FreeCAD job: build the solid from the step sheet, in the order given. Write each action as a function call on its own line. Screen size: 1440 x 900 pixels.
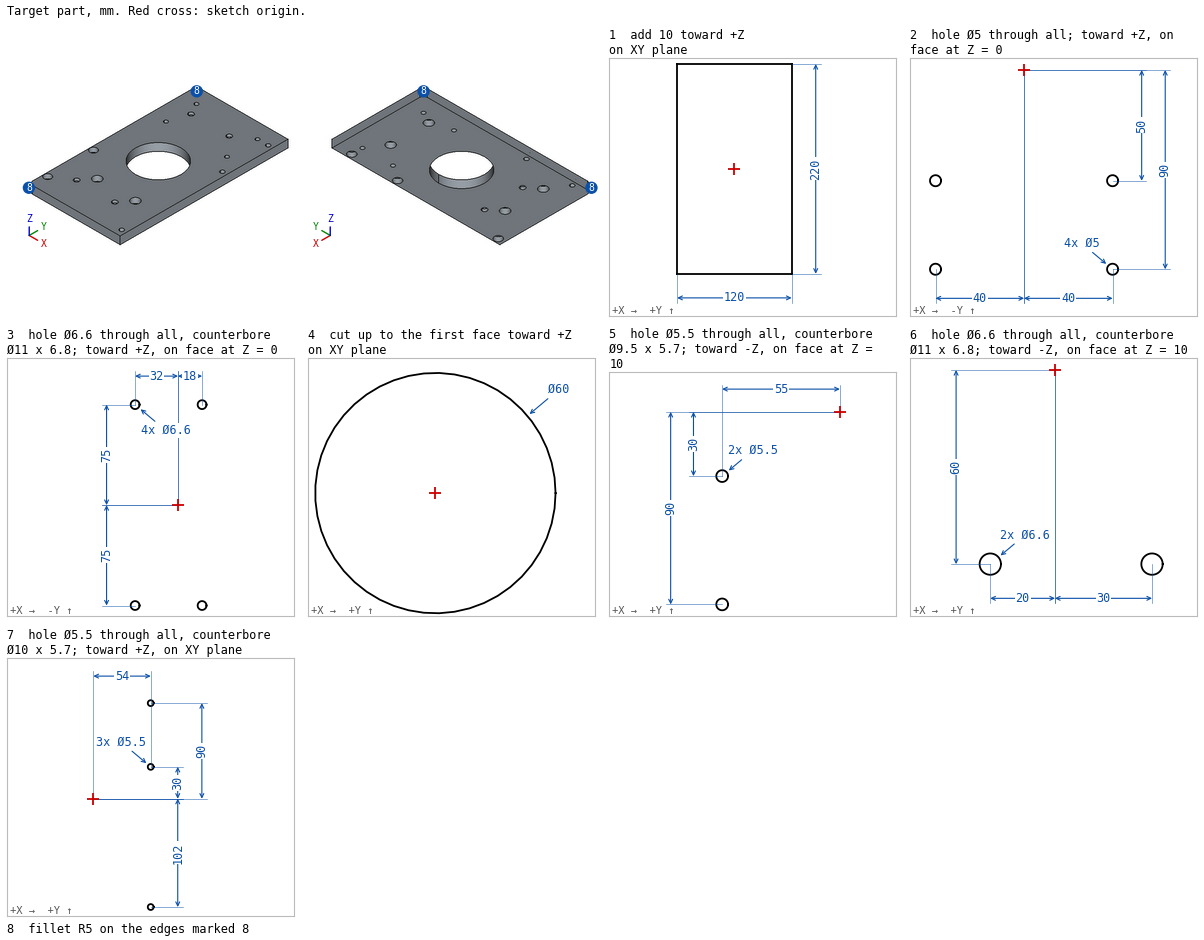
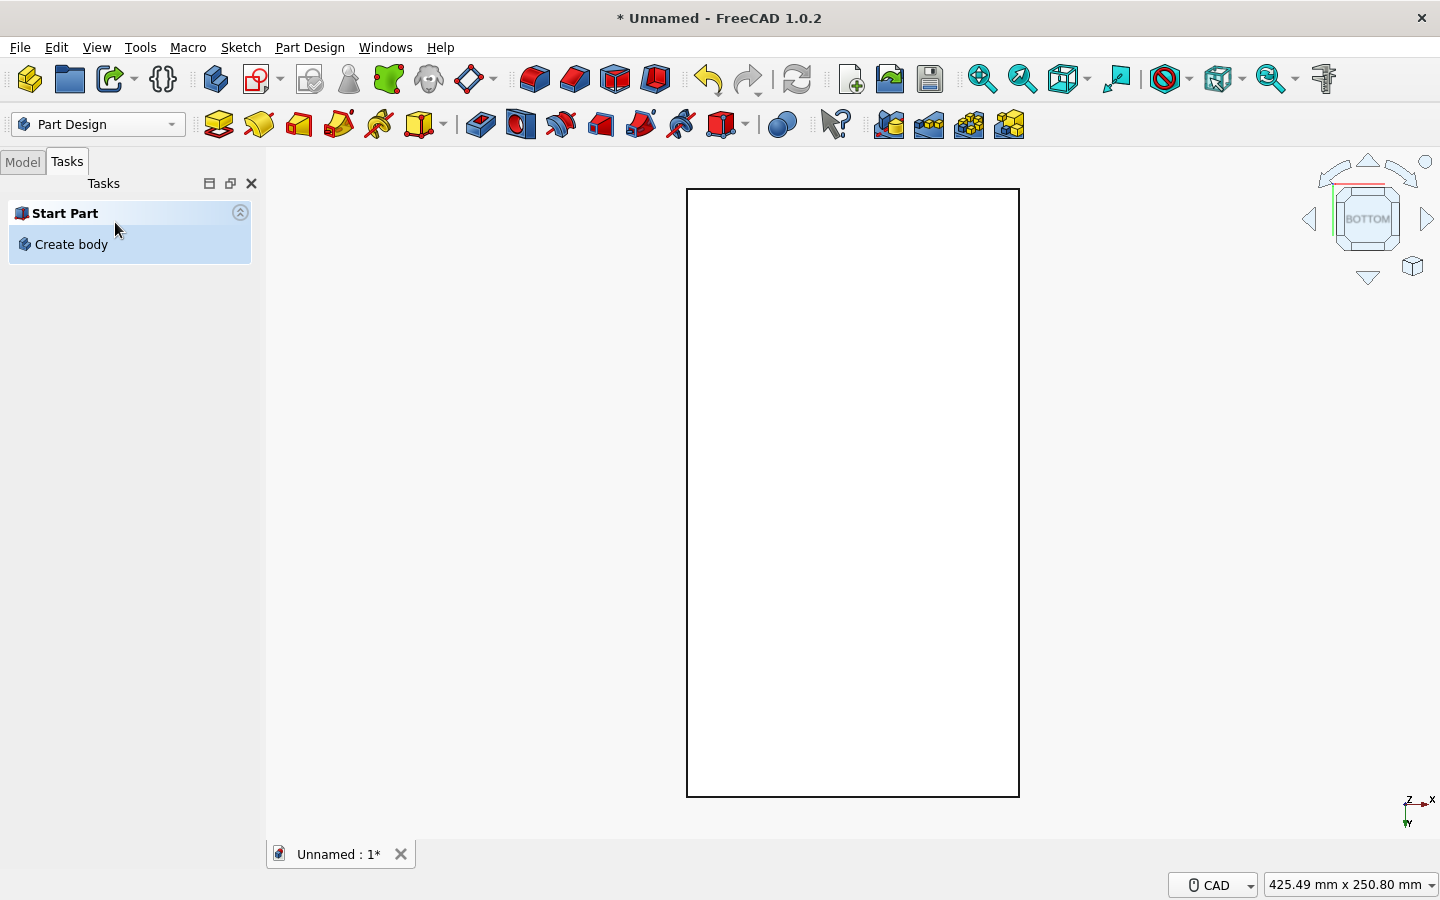
click(853, 579)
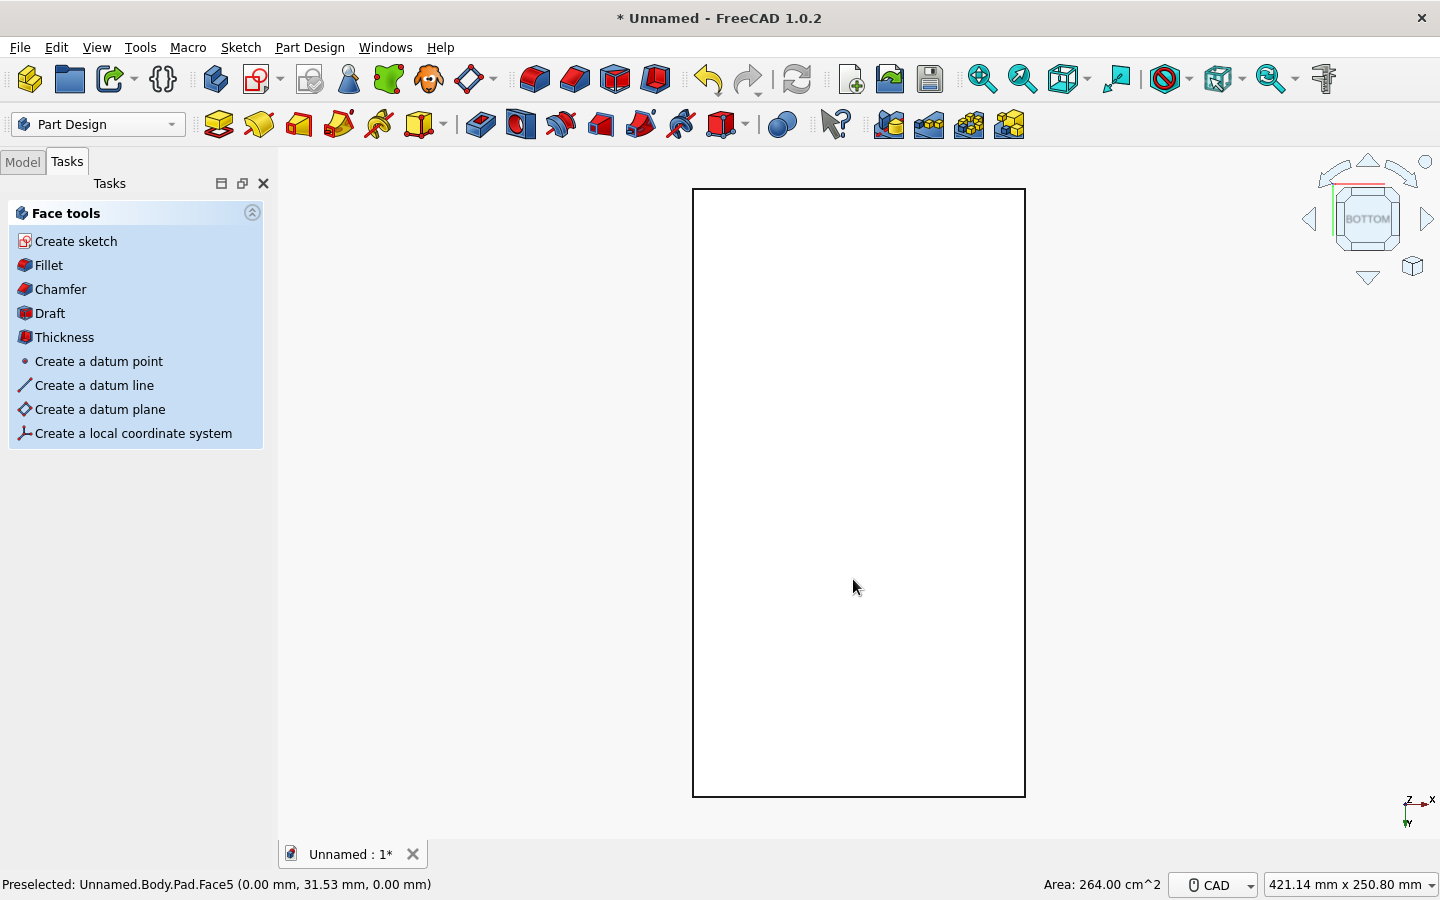
click(256, 80)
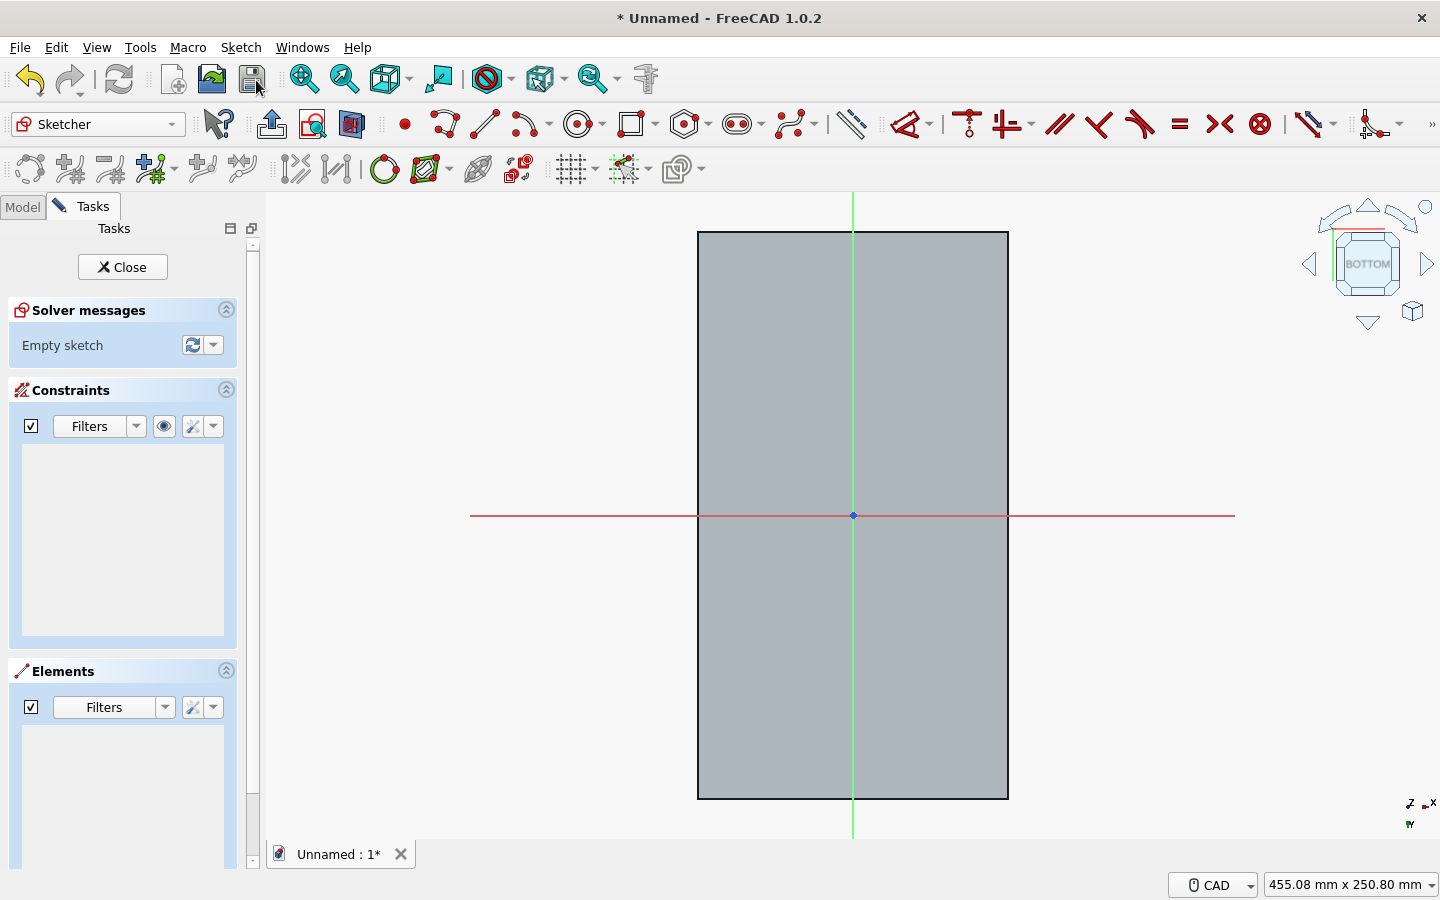
scroll(936, 780, up, 3)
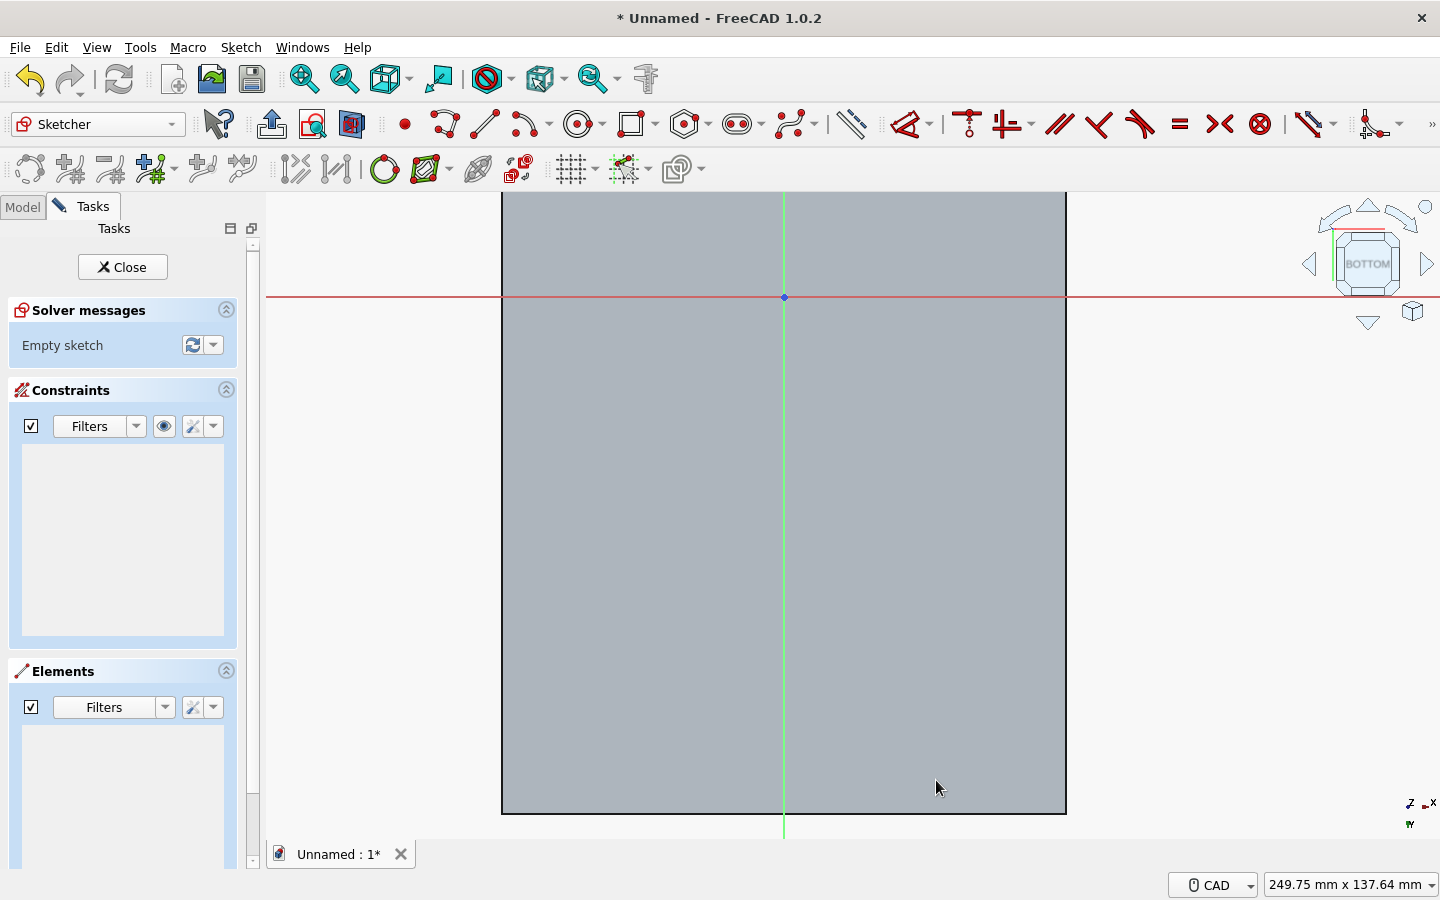
key(g)
key(c)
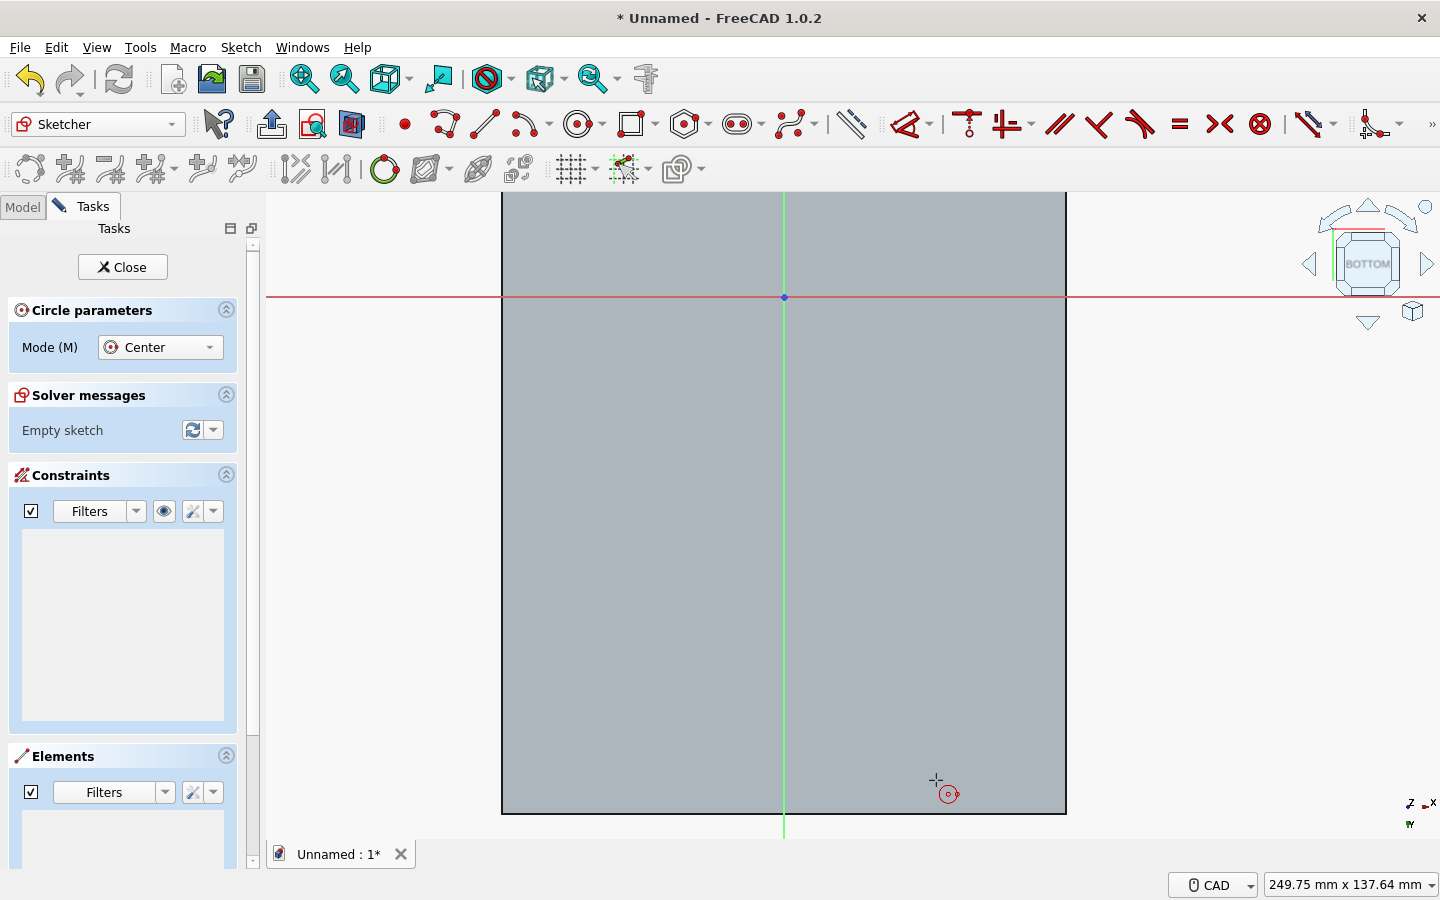
scroll(972, 720, up, 4)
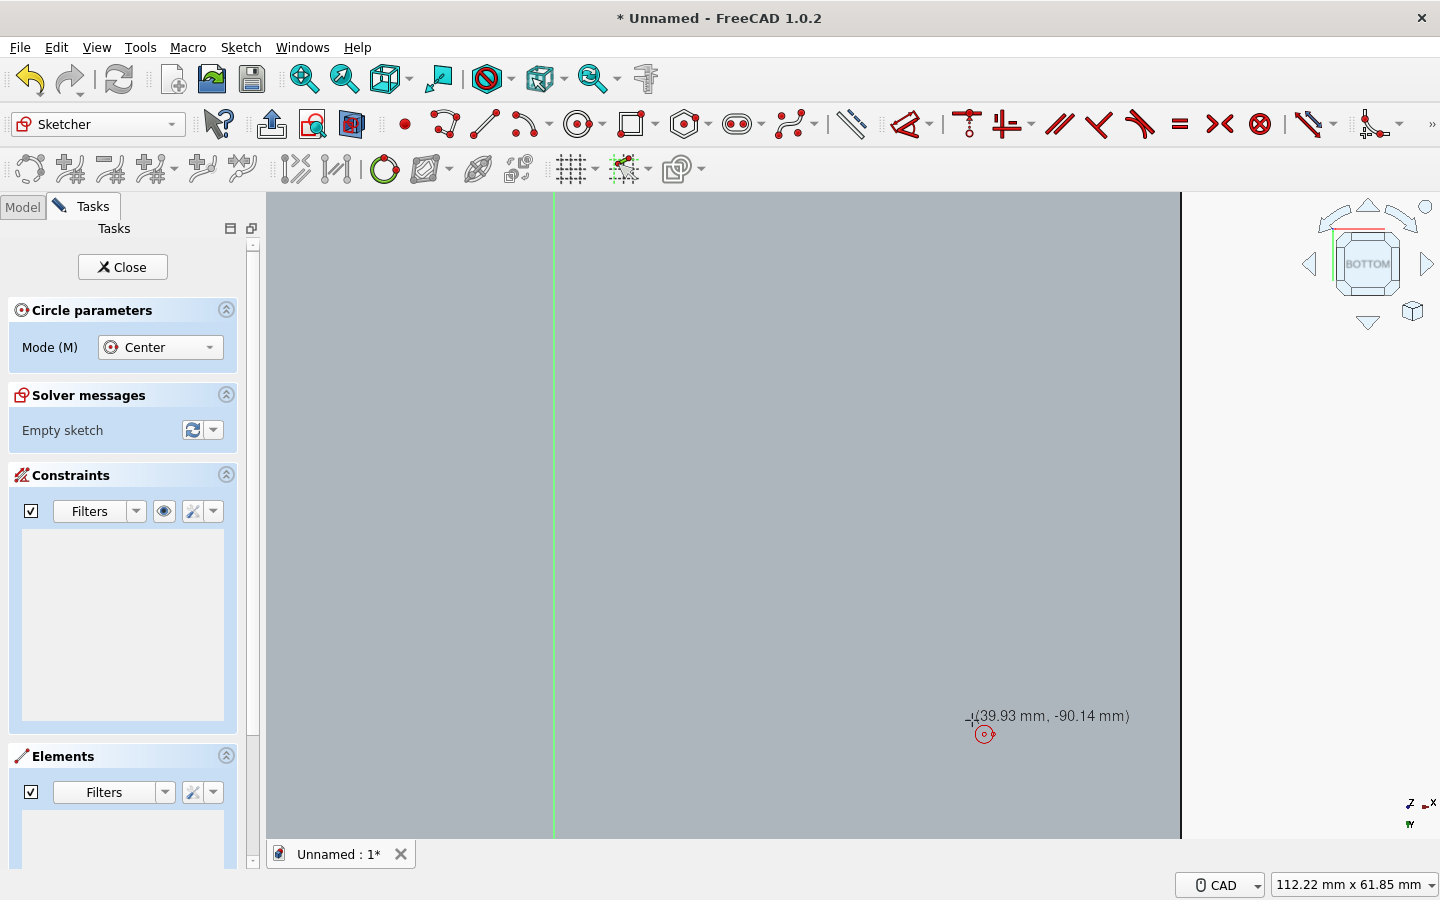
click(972, 720)
move(990, 701)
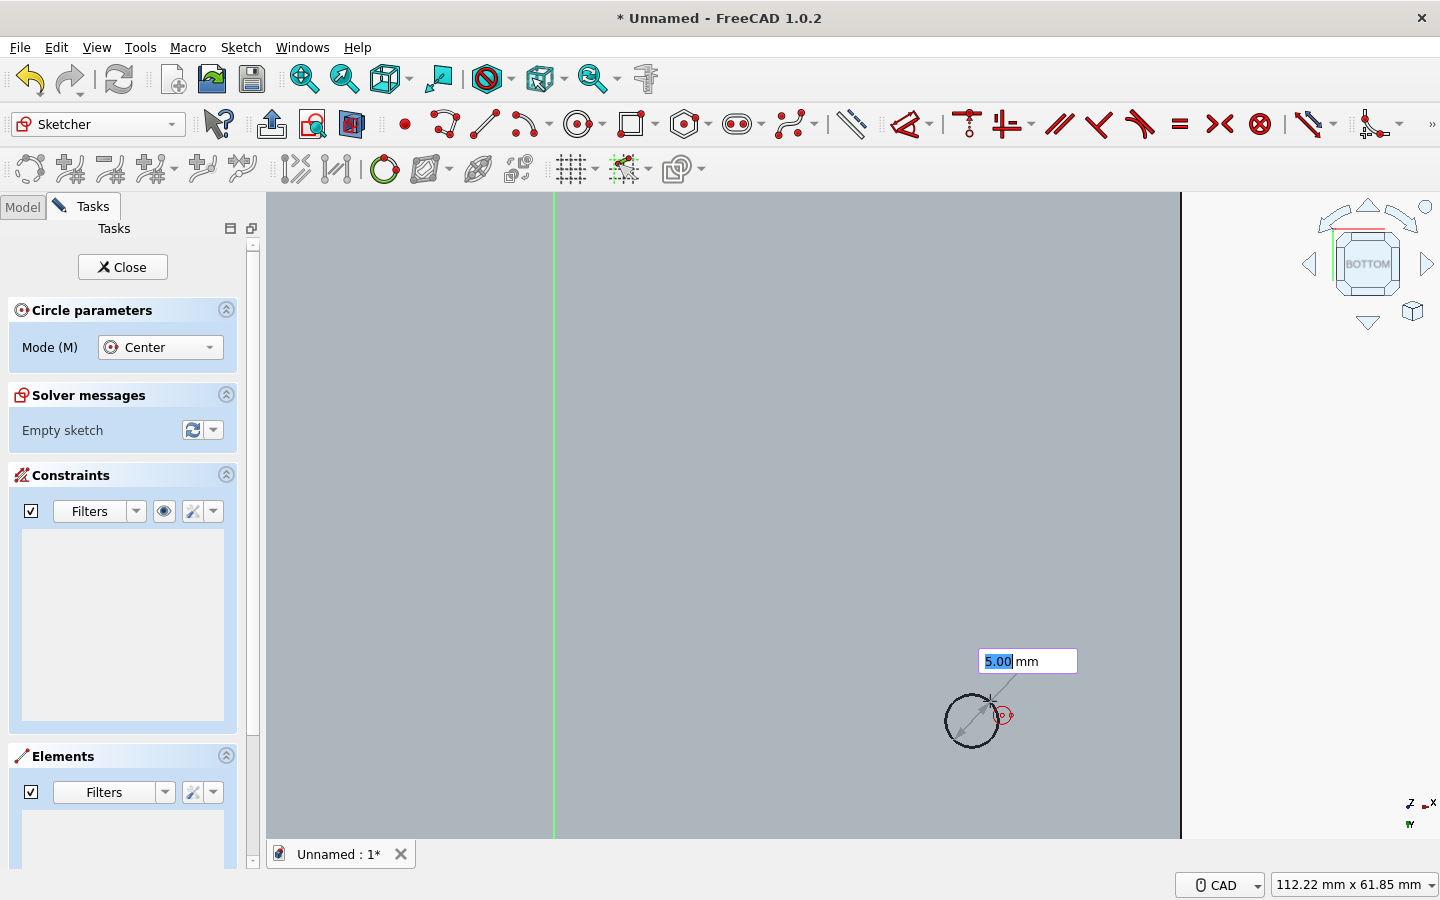
text(5)
key(Return)